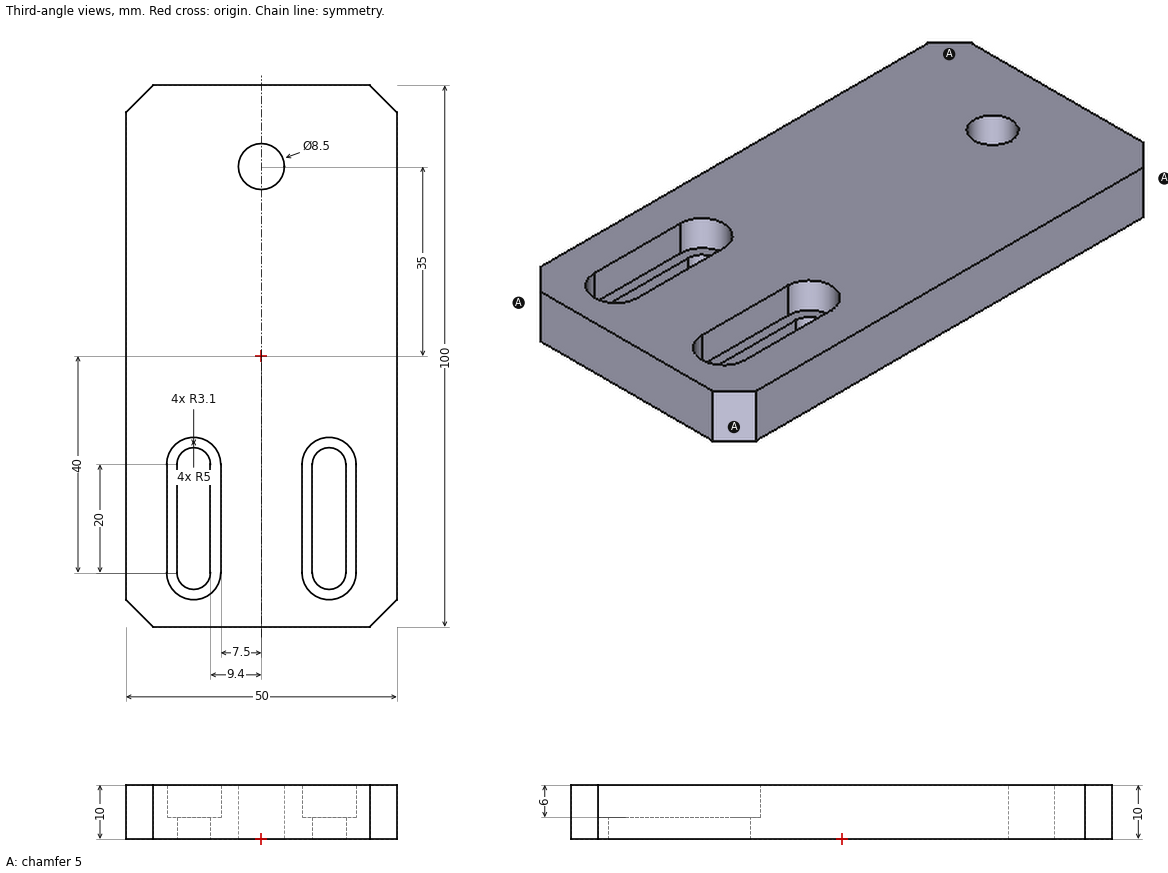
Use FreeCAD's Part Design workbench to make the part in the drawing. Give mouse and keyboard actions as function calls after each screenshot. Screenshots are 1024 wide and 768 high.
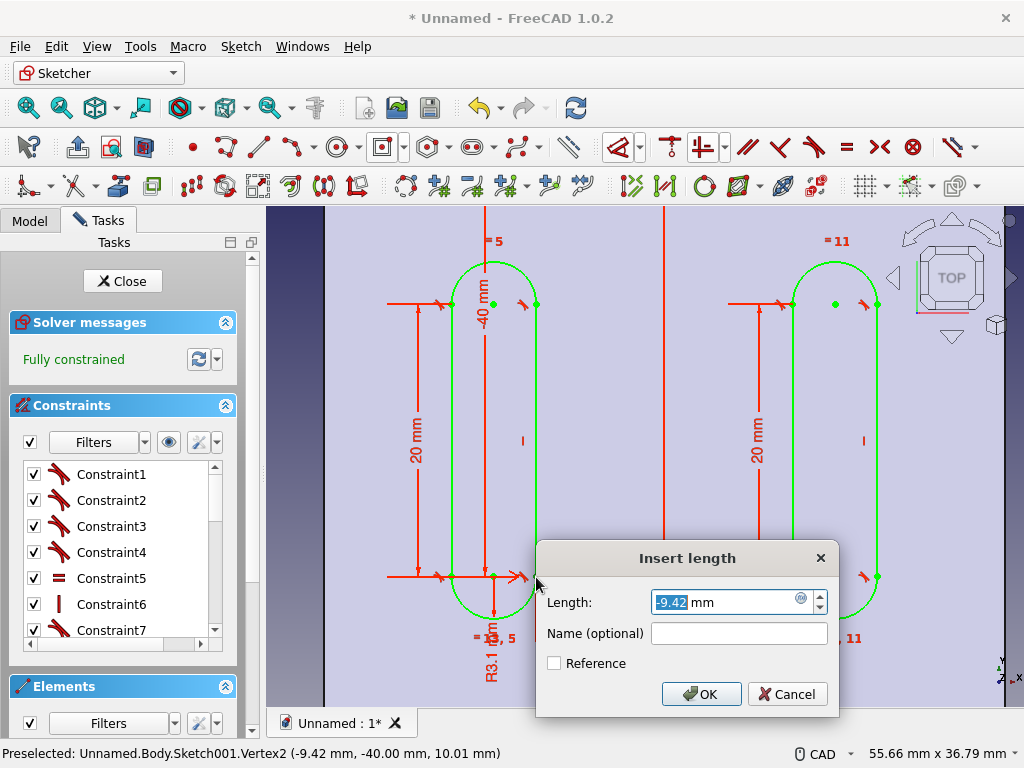
text(-9.4)
key(Return)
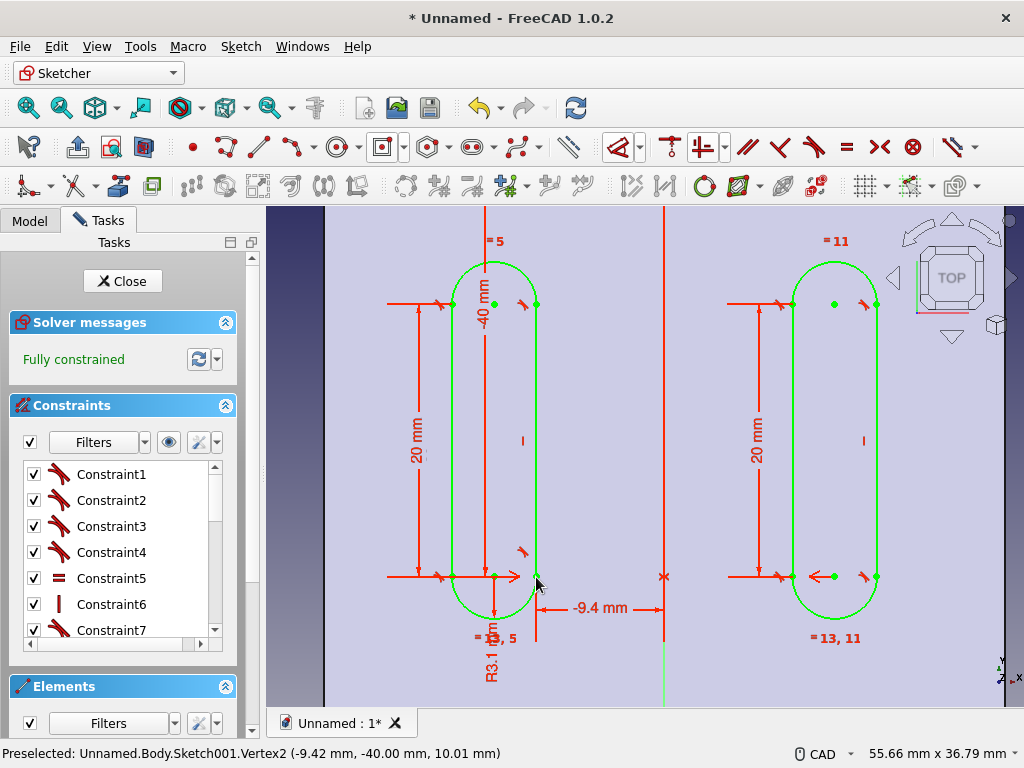
click(123, 281)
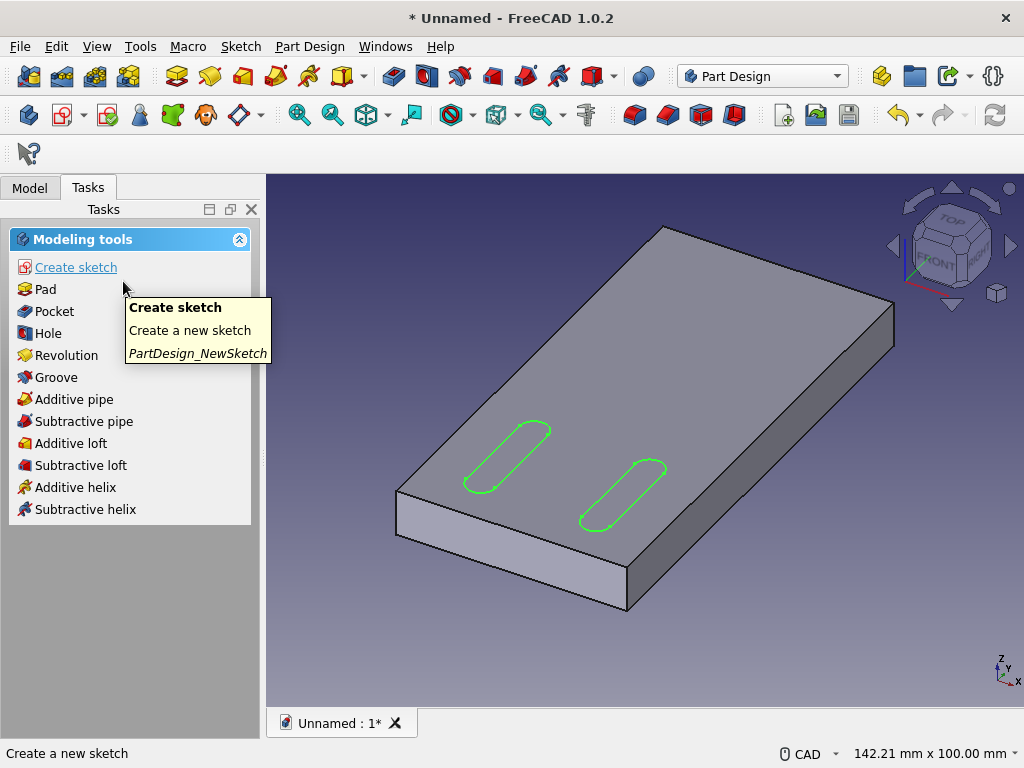
click(394, 76)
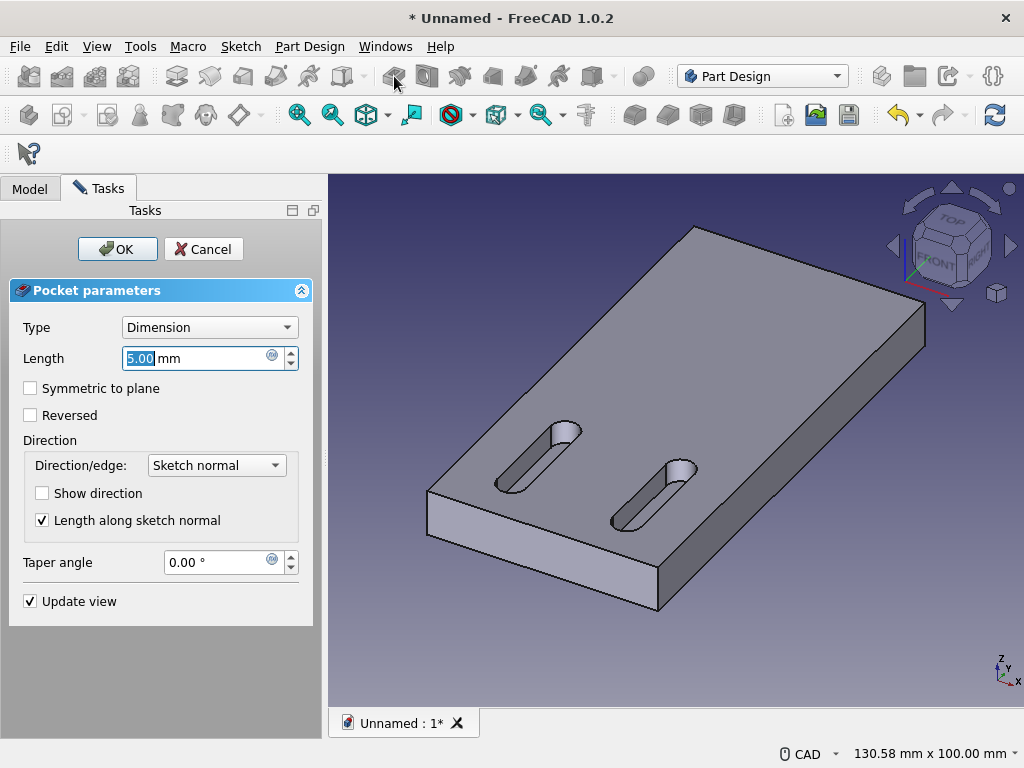
text(10)
key(Tab)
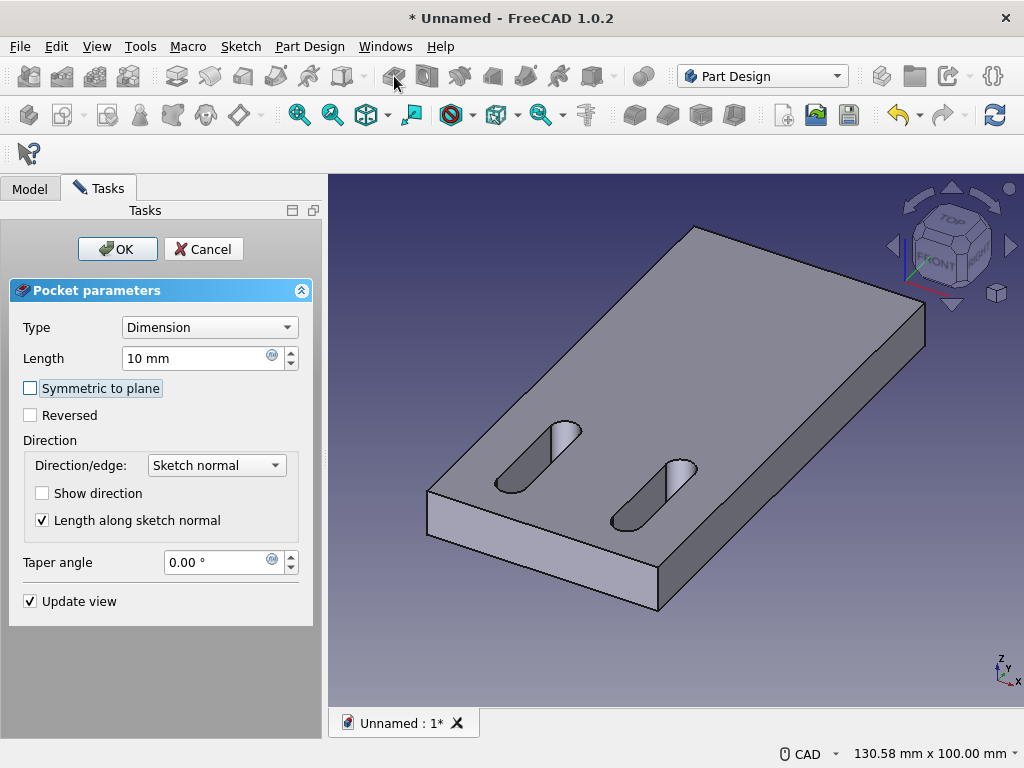
click(118, 249)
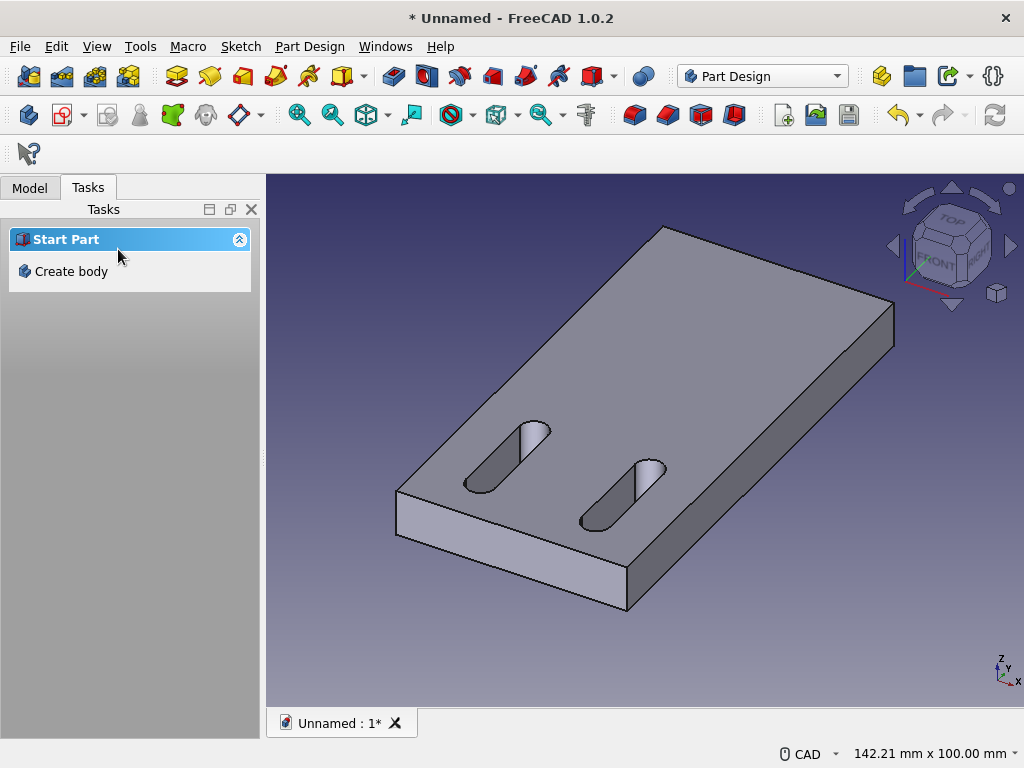
click(683, 358)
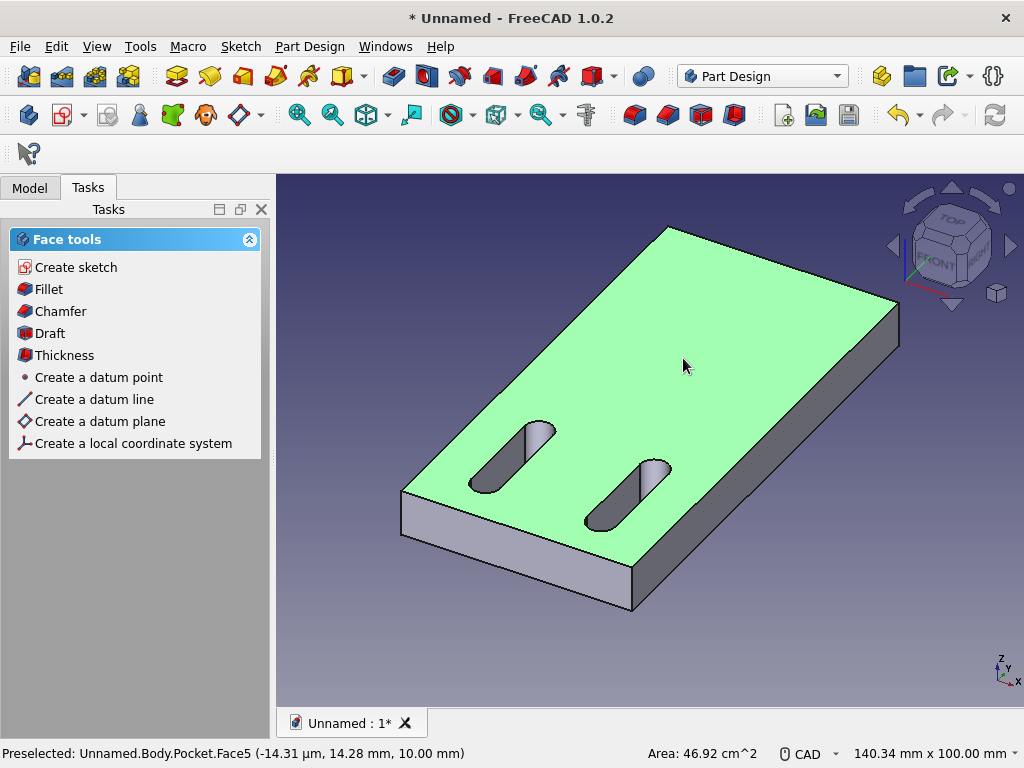
click(62, 116)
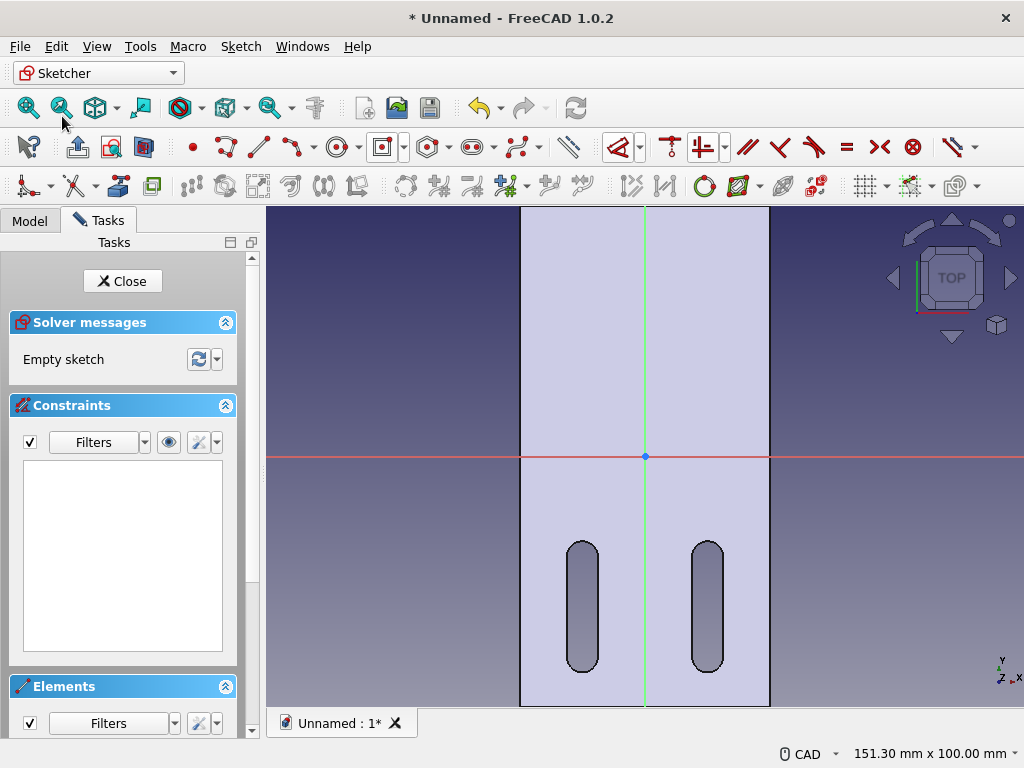
scroll(294, 234, down, 1)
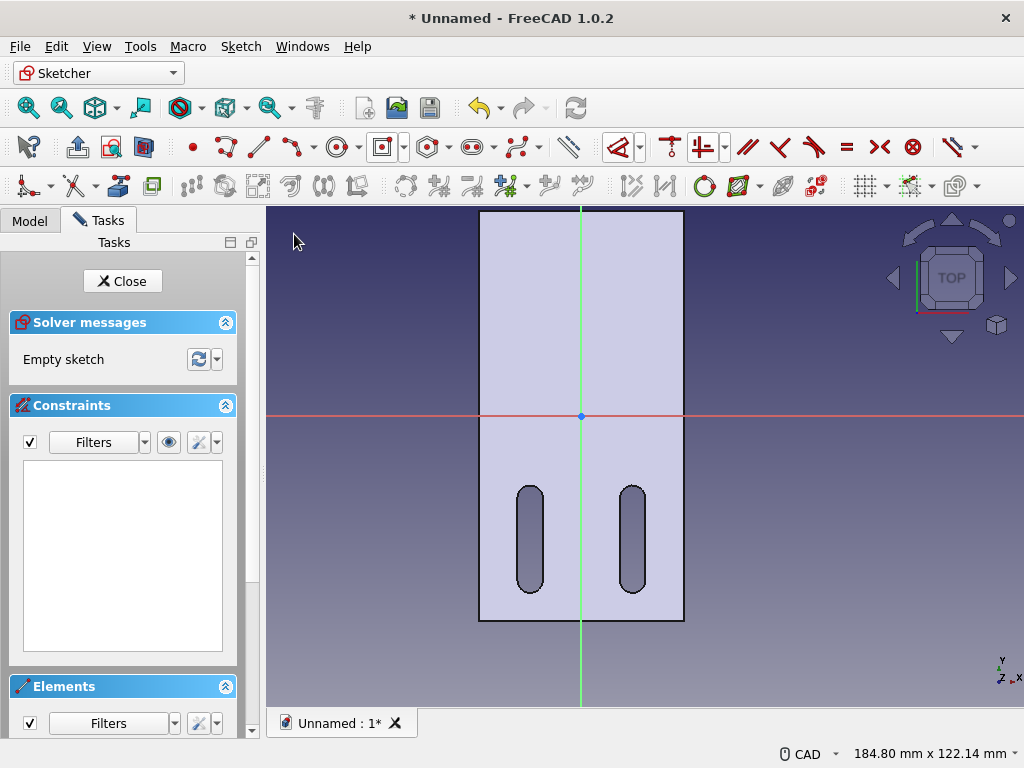
scroll(587, 572, up, 3)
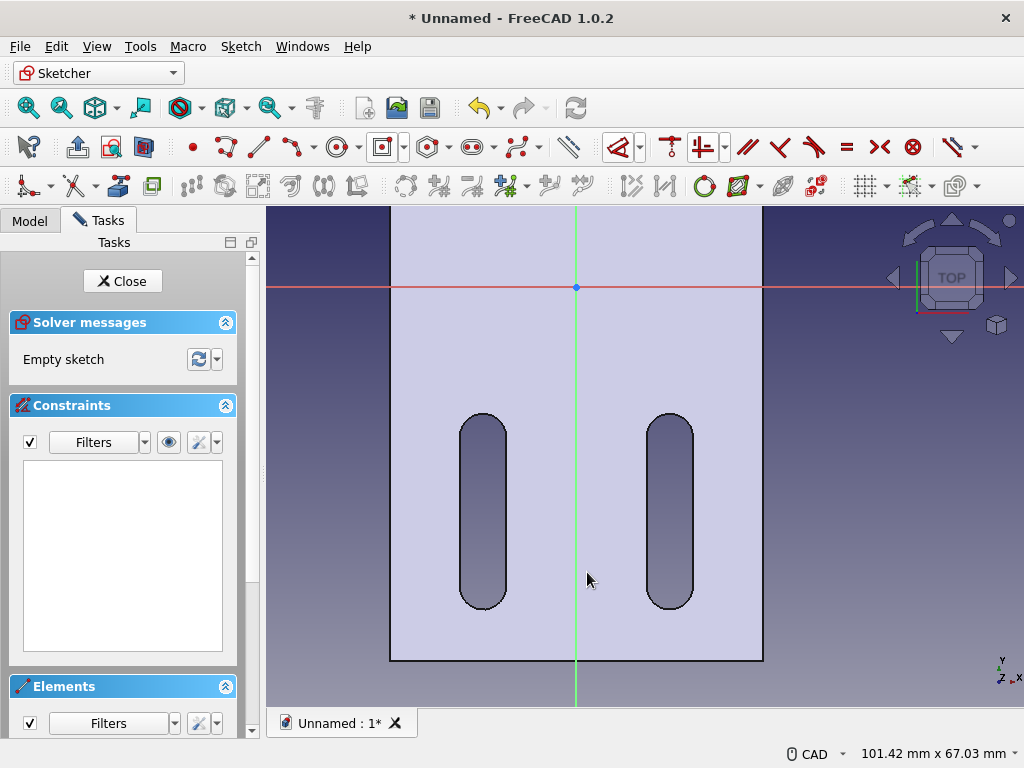
click(472, 148)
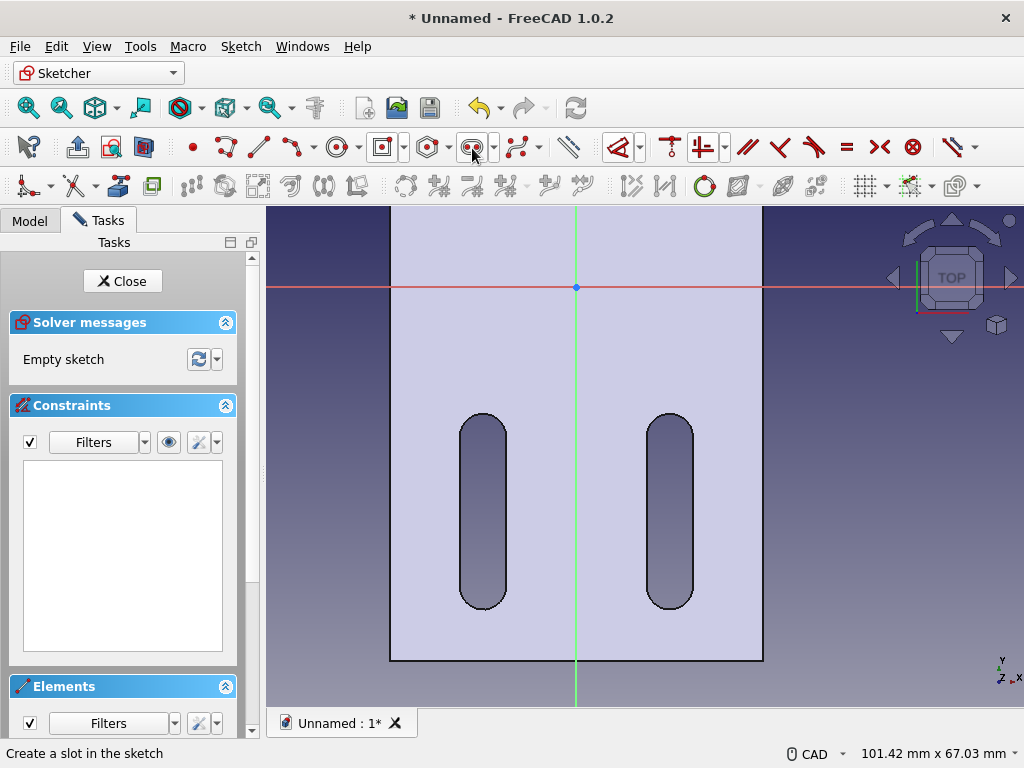
click(483, 586)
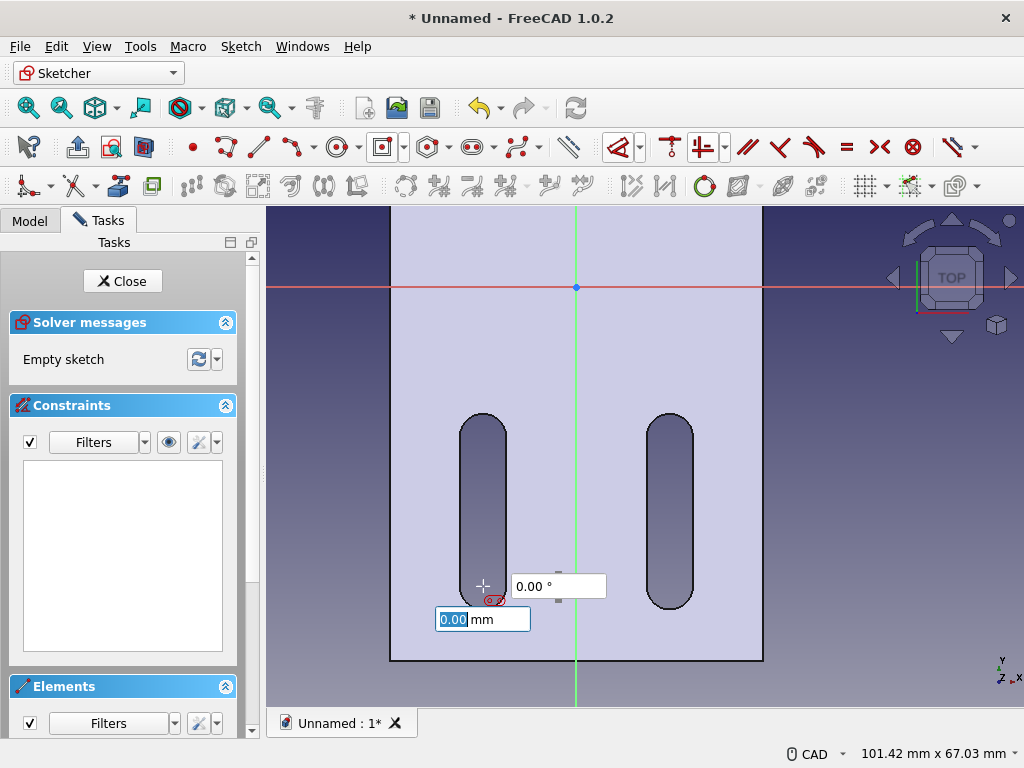
click(483, 437)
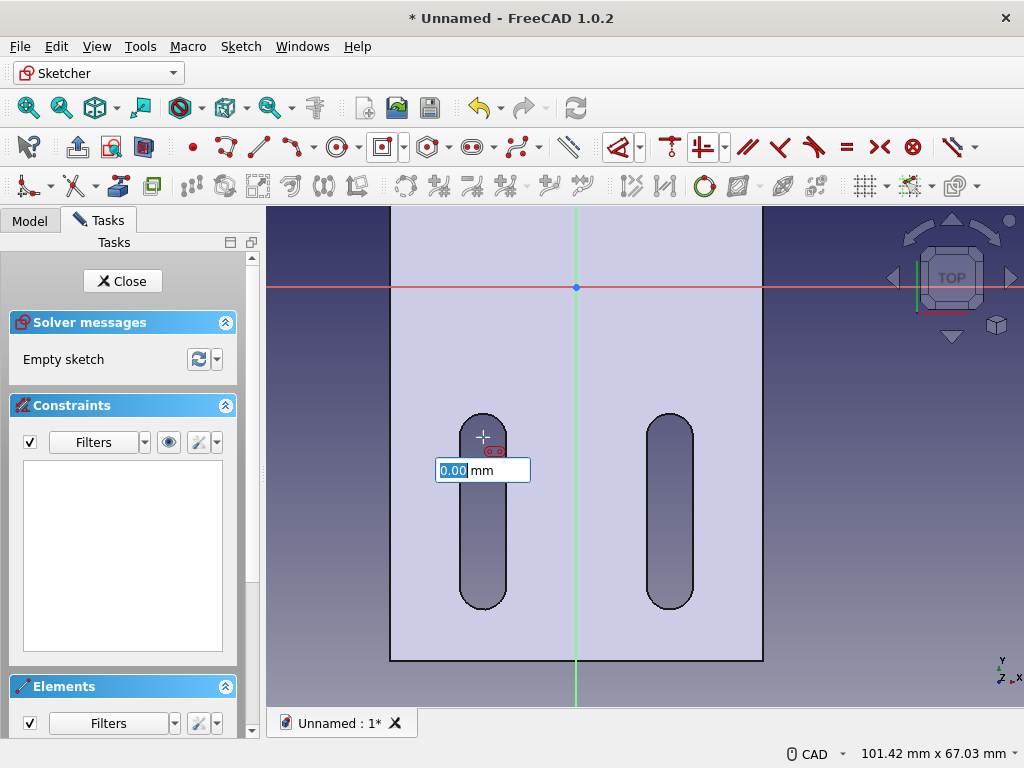
click(520, 512)